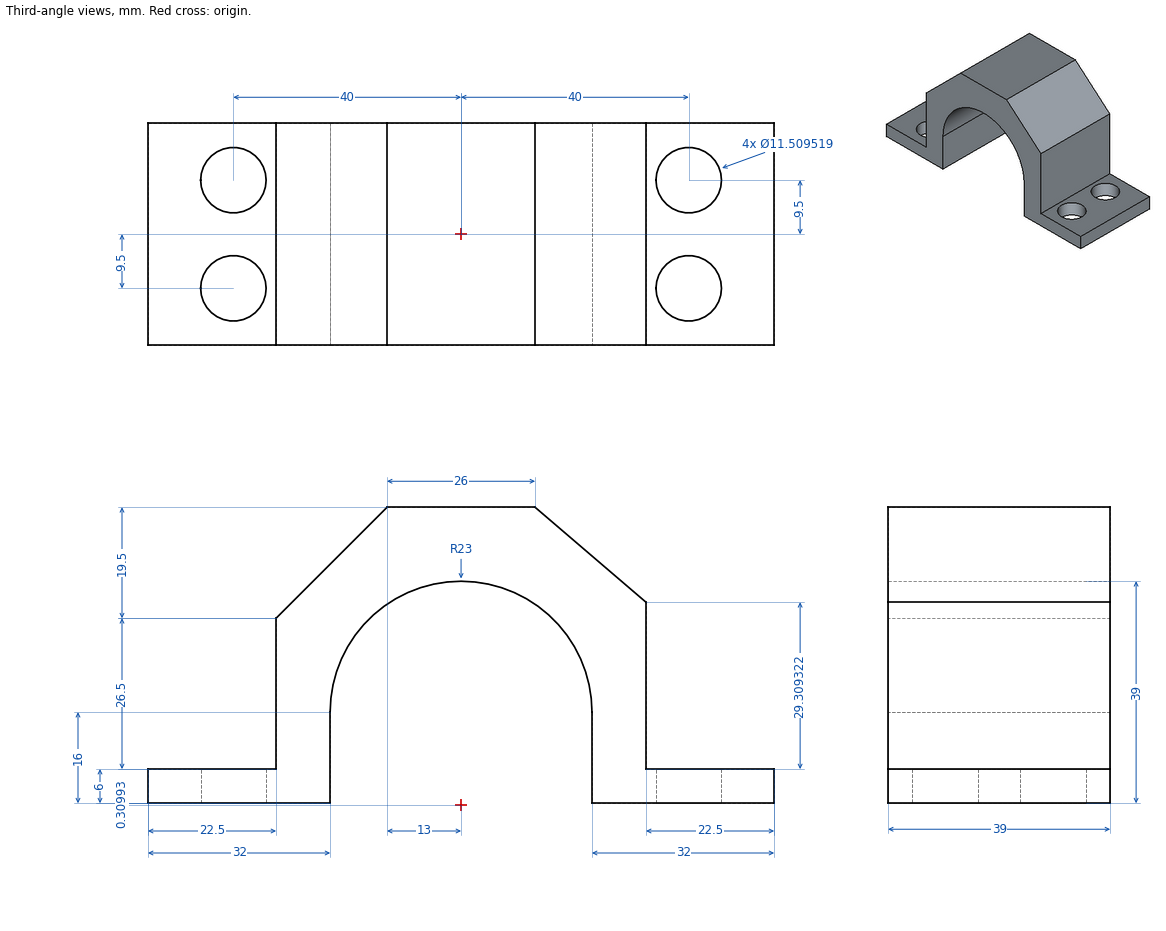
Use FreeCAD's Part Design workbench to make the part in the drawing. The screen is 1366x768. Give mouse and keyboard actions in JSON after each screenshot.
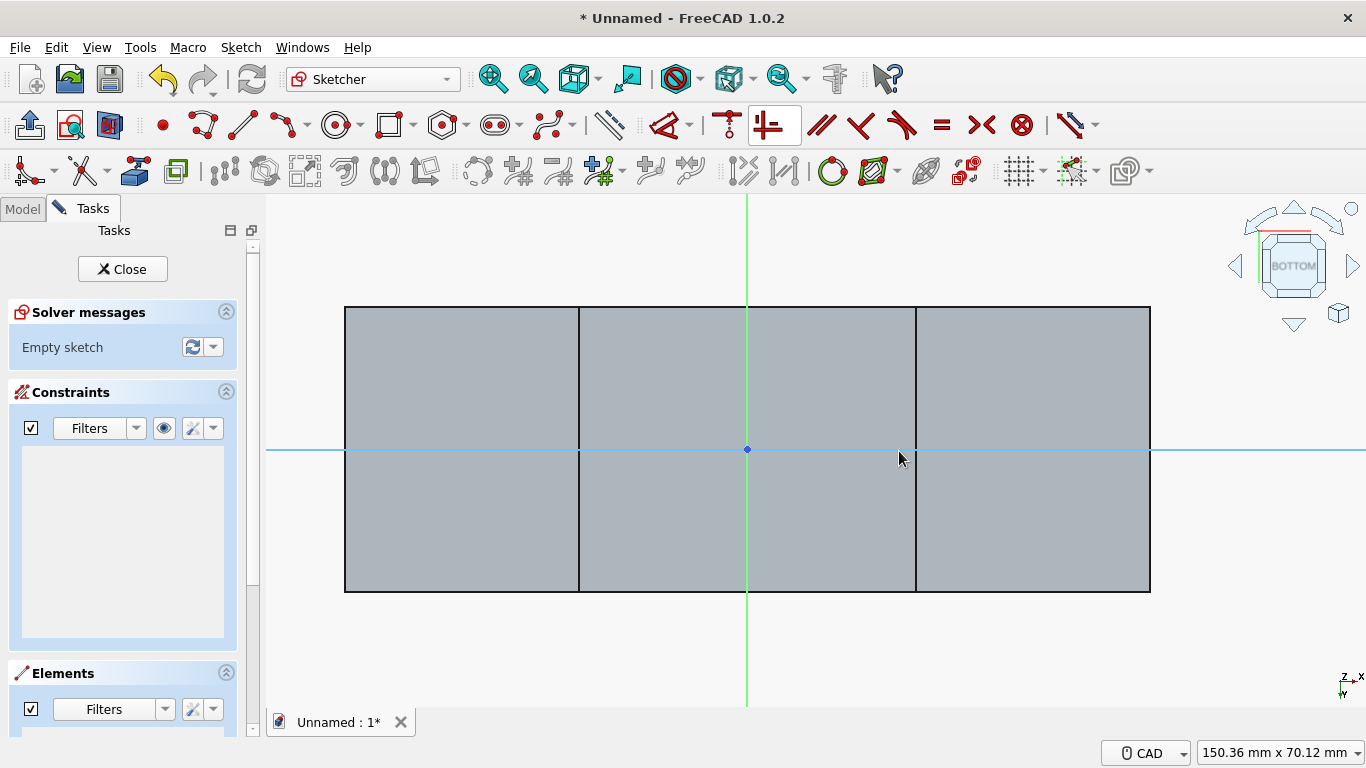
{"action": "left_click", "coordinate": [336, 126]}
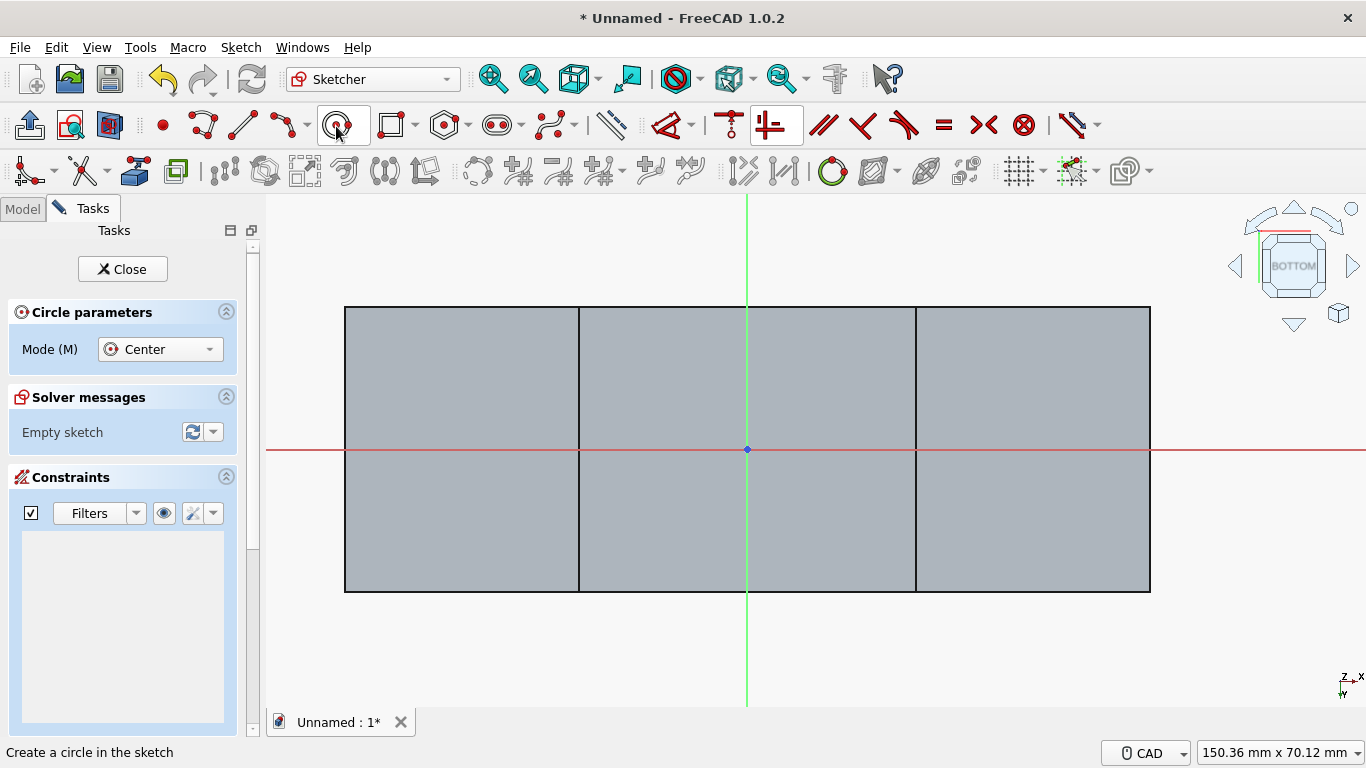
{"action": "left_click", "coordinate": [1040, 519]}
{"action": "left_click", "coordinate": [1070, 489]}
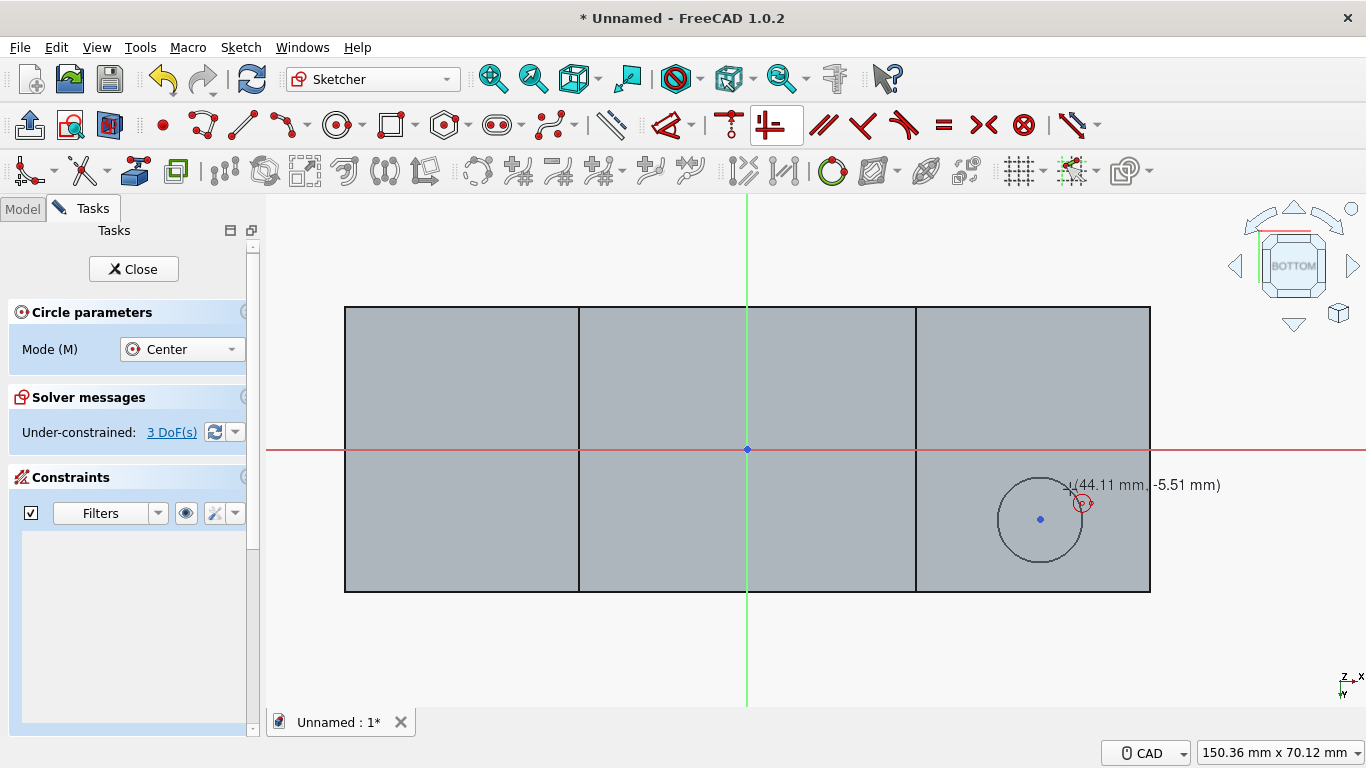
{"action": "left_click", "coordinate": [455, 519]}
{"action": "left_click", "coordinate": [484, 489]}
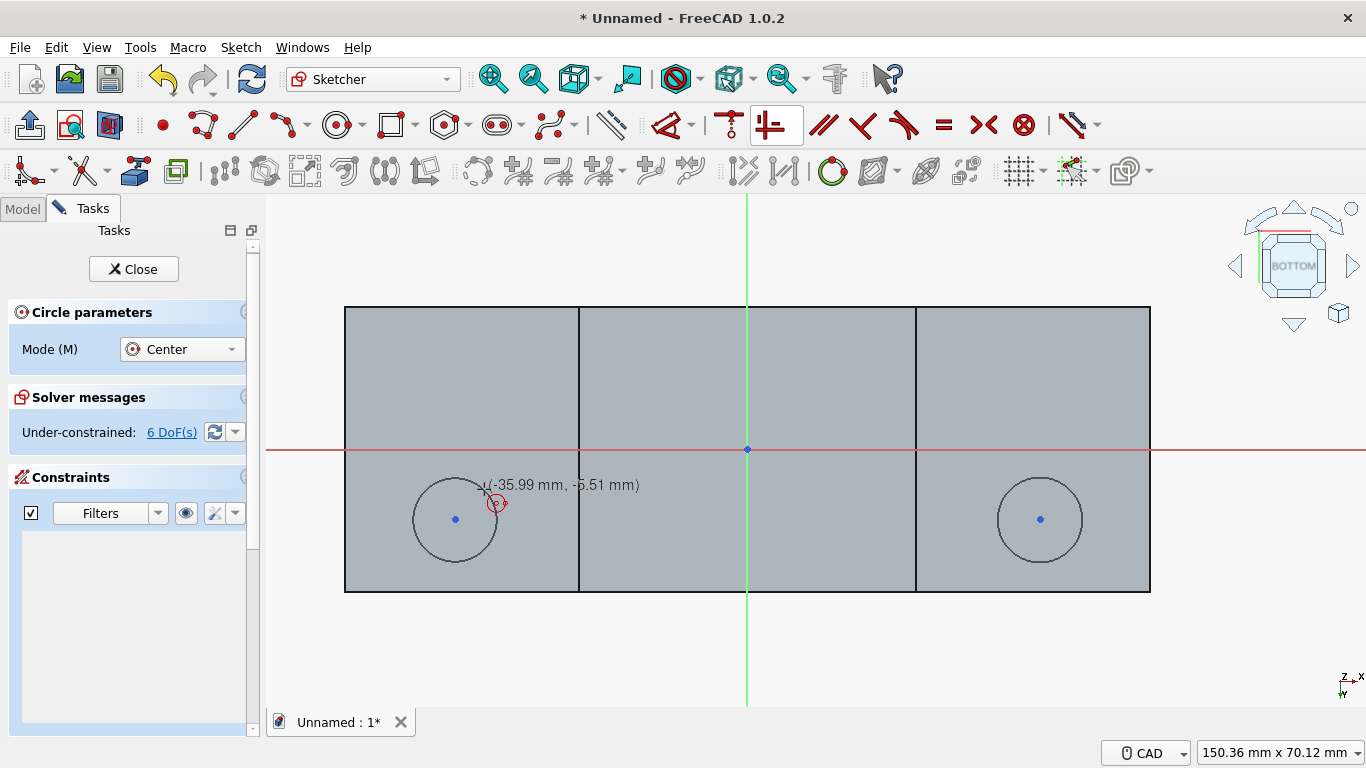
{"action": "left_click", "coordinate": [455, 380]}
{"action": "left_click", "coordinate": [484, 350]}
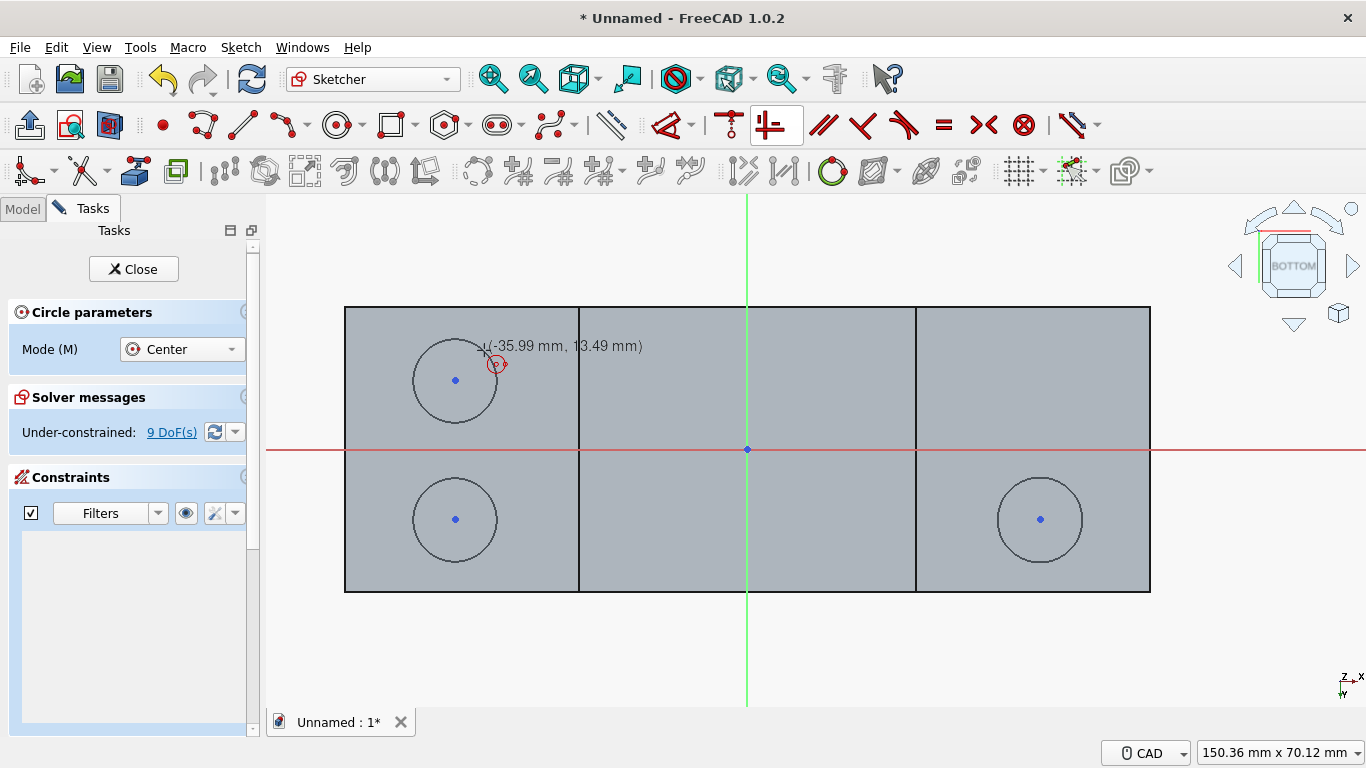
{"action": "left_click", "coordinate": [1040, 380]}
{"action": "left_click", "coordinate": [1070, 350]}
{"action": "key", "text": "Escape"}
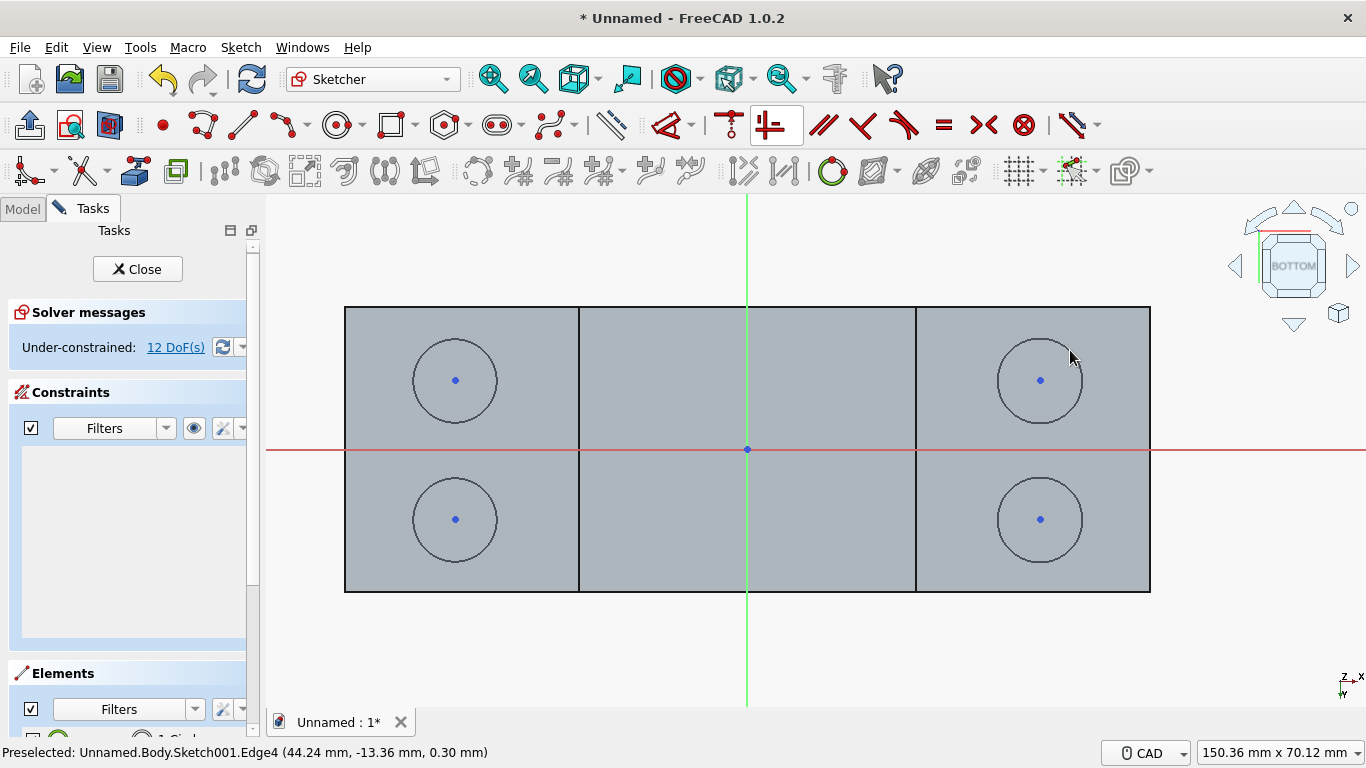
{"action": "left_click", "coordinate": [1070, 490]}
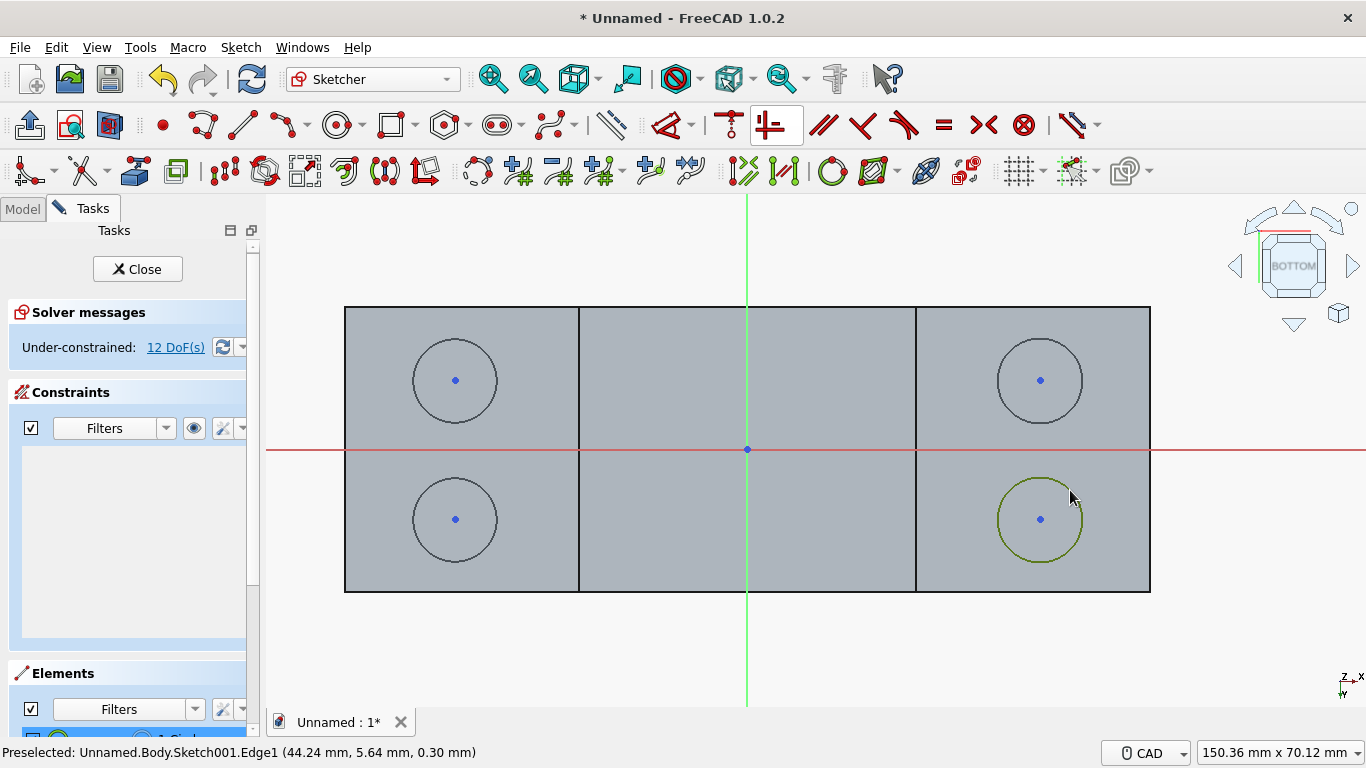
{"action": "left_click", "coordinate": [484, 490]}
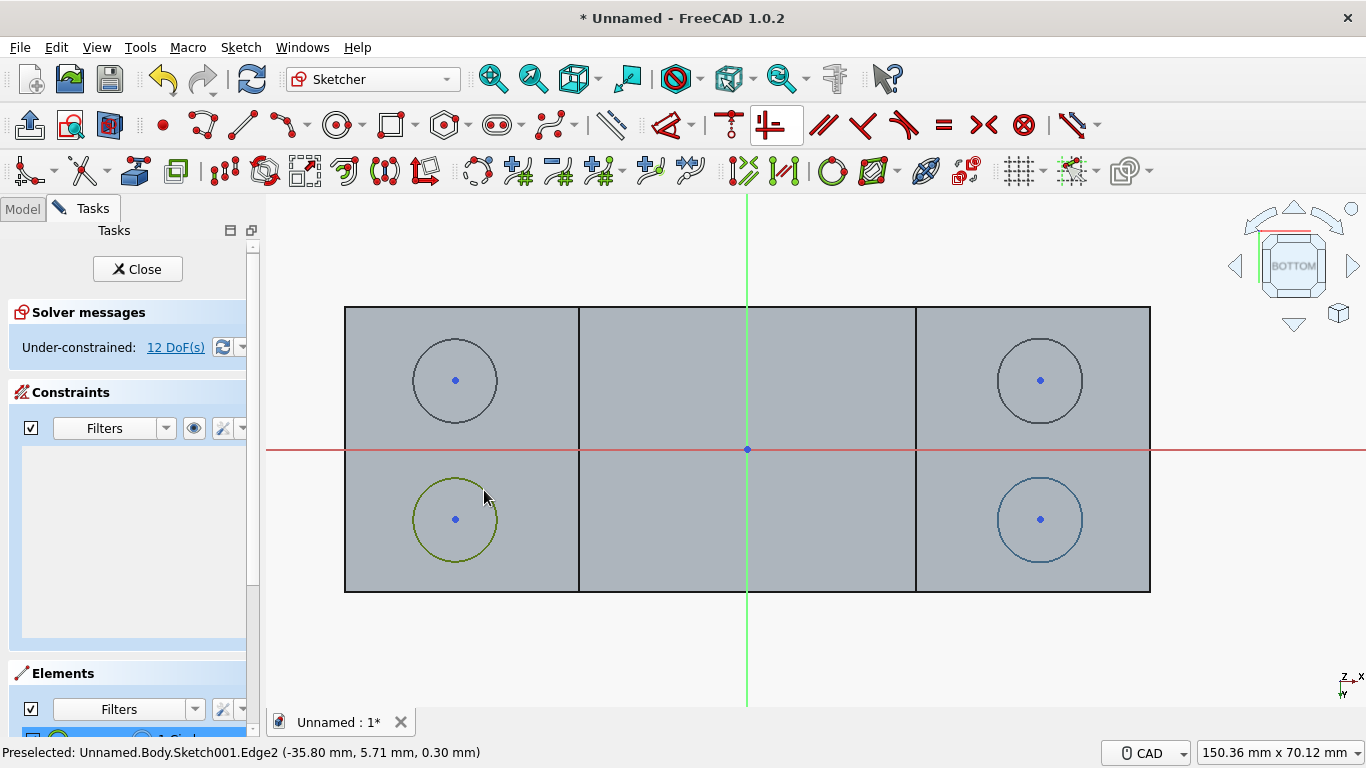
{"action": "left_click", "coordinate": [484, 351]}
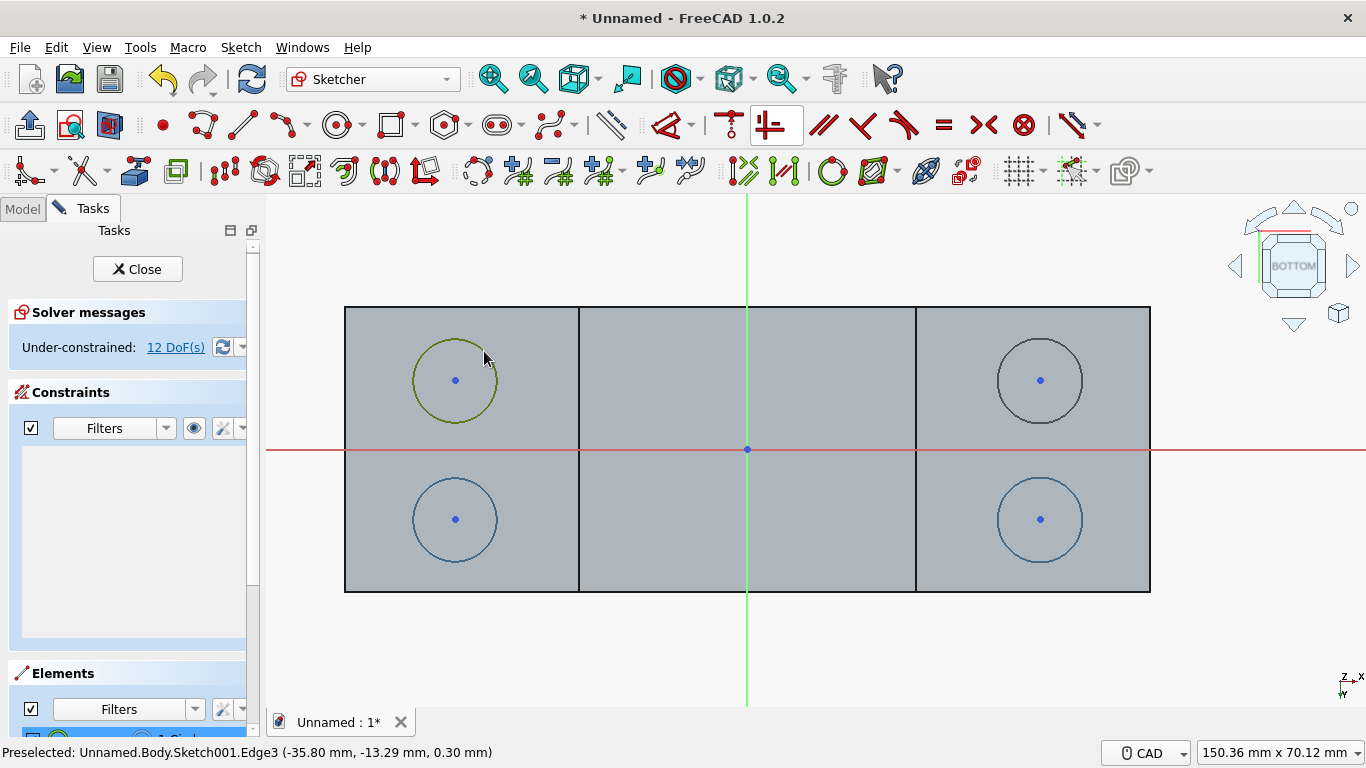
{"action": "left_click", "coordinate": [1070, 351]}